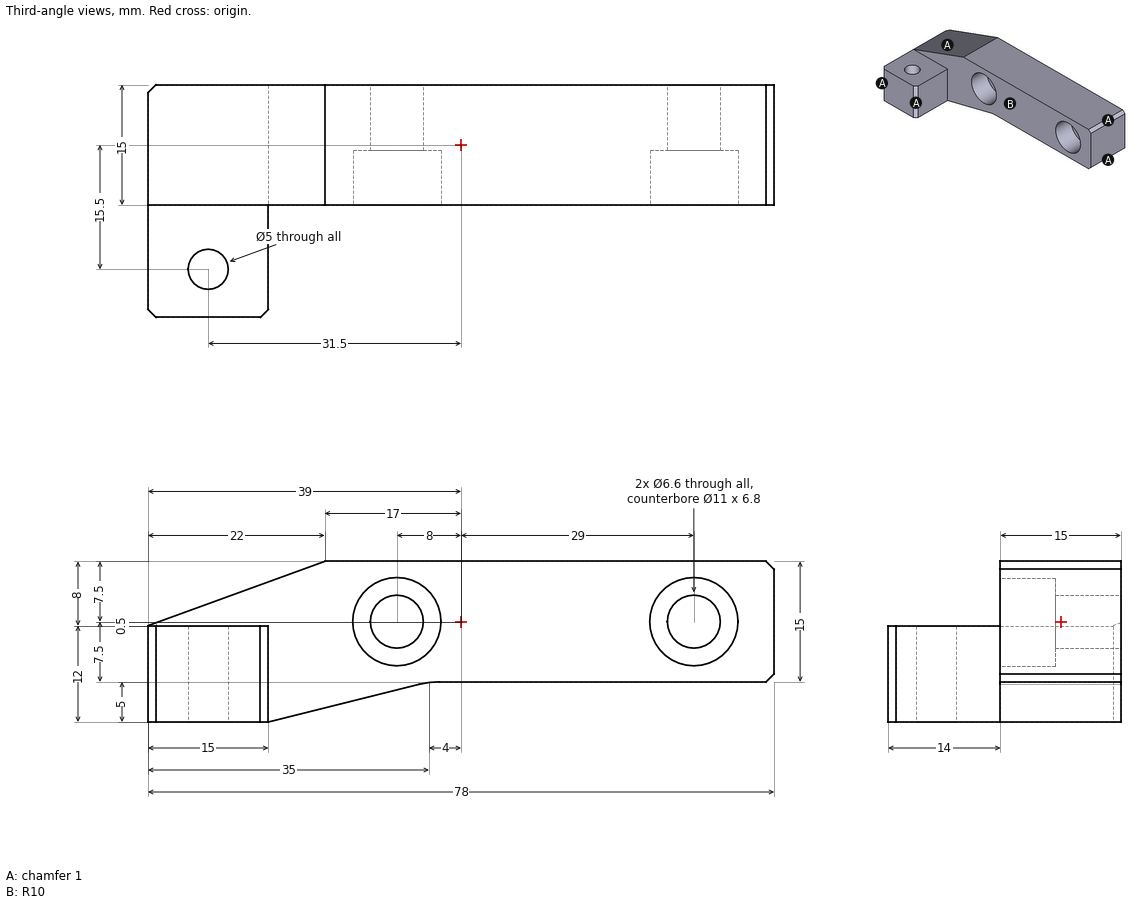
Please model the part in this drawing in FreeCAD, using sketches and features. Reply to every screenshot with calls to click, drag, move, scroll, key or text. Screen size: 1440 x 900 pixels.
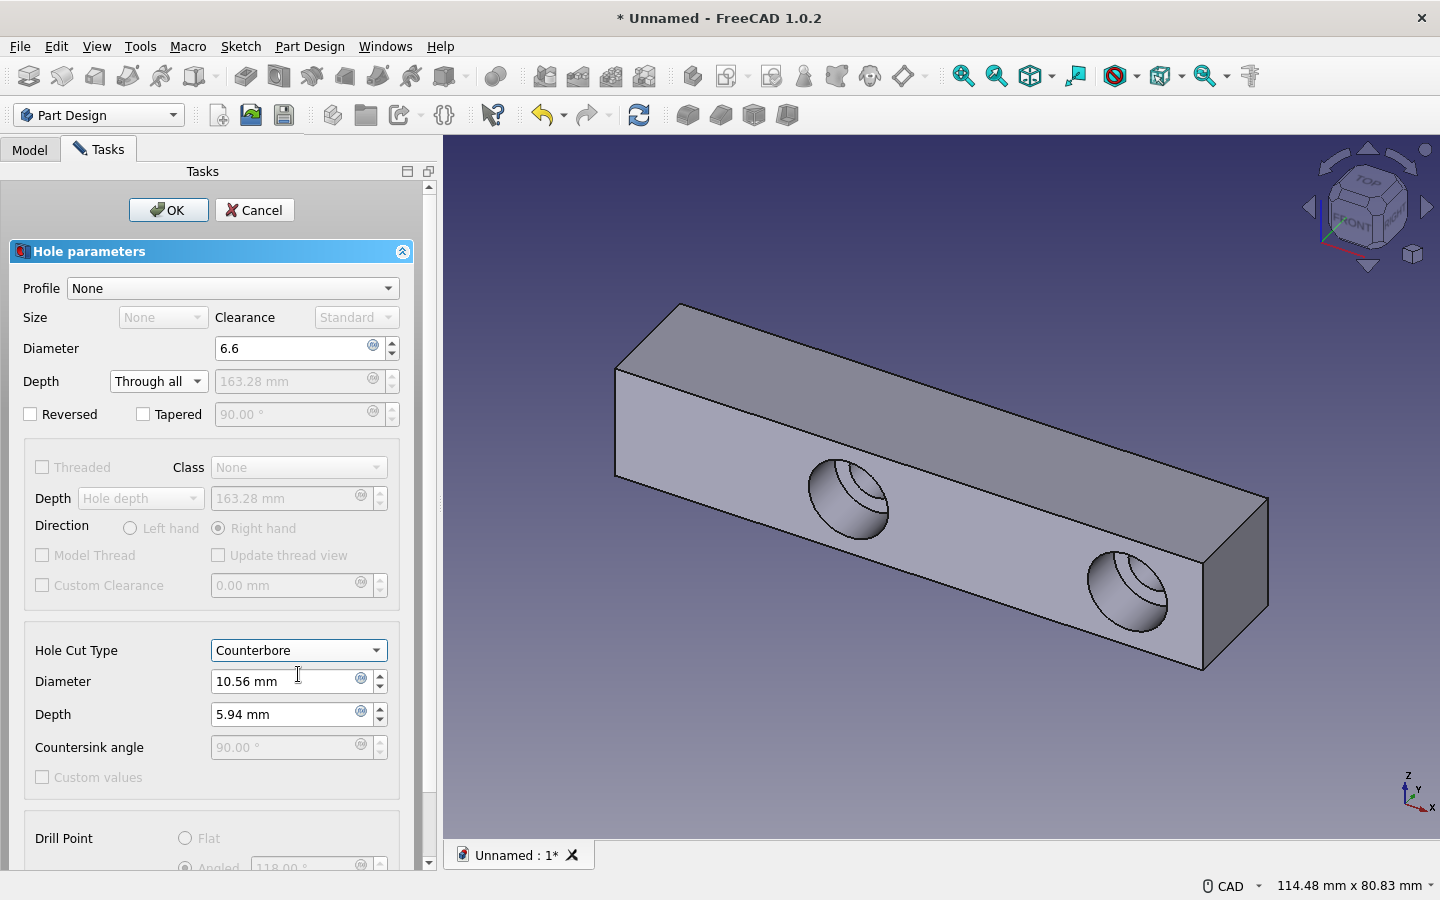
triple_click(292, 682)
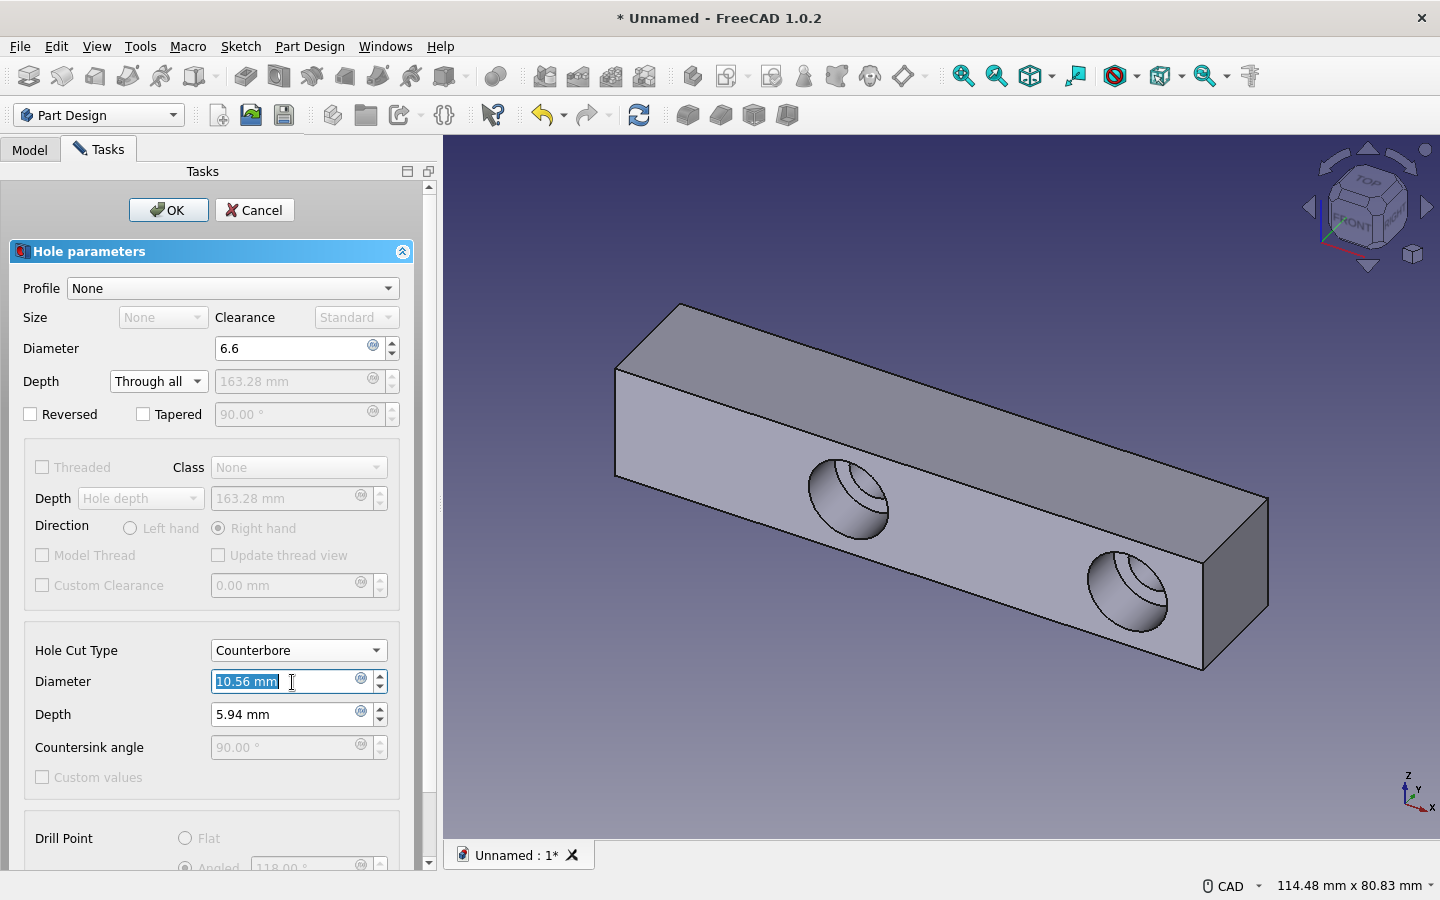
text(11)
key(Tab)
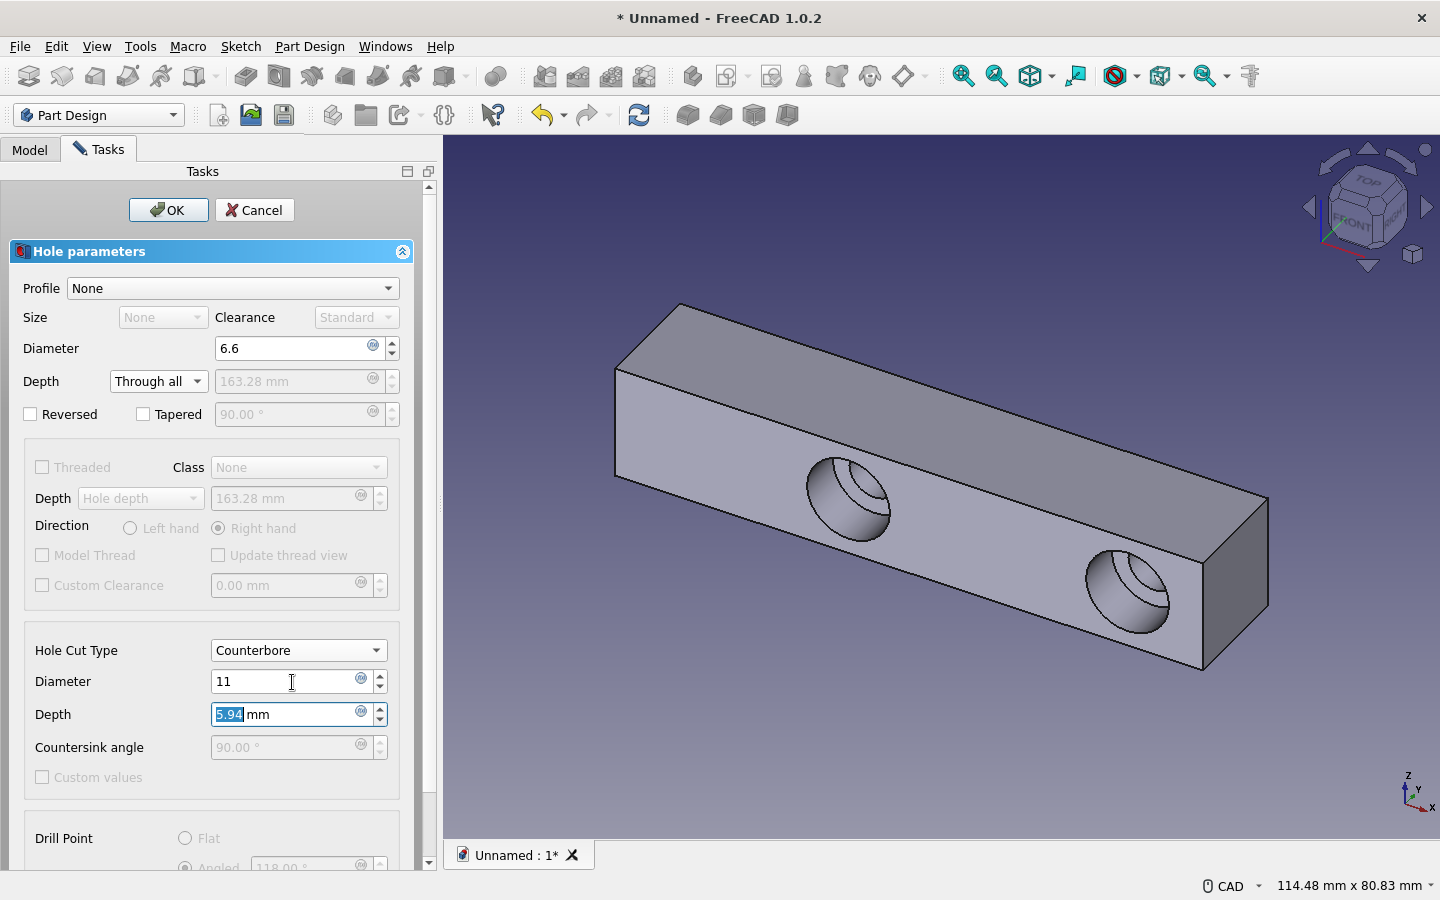
text(6.8)
key(Tab)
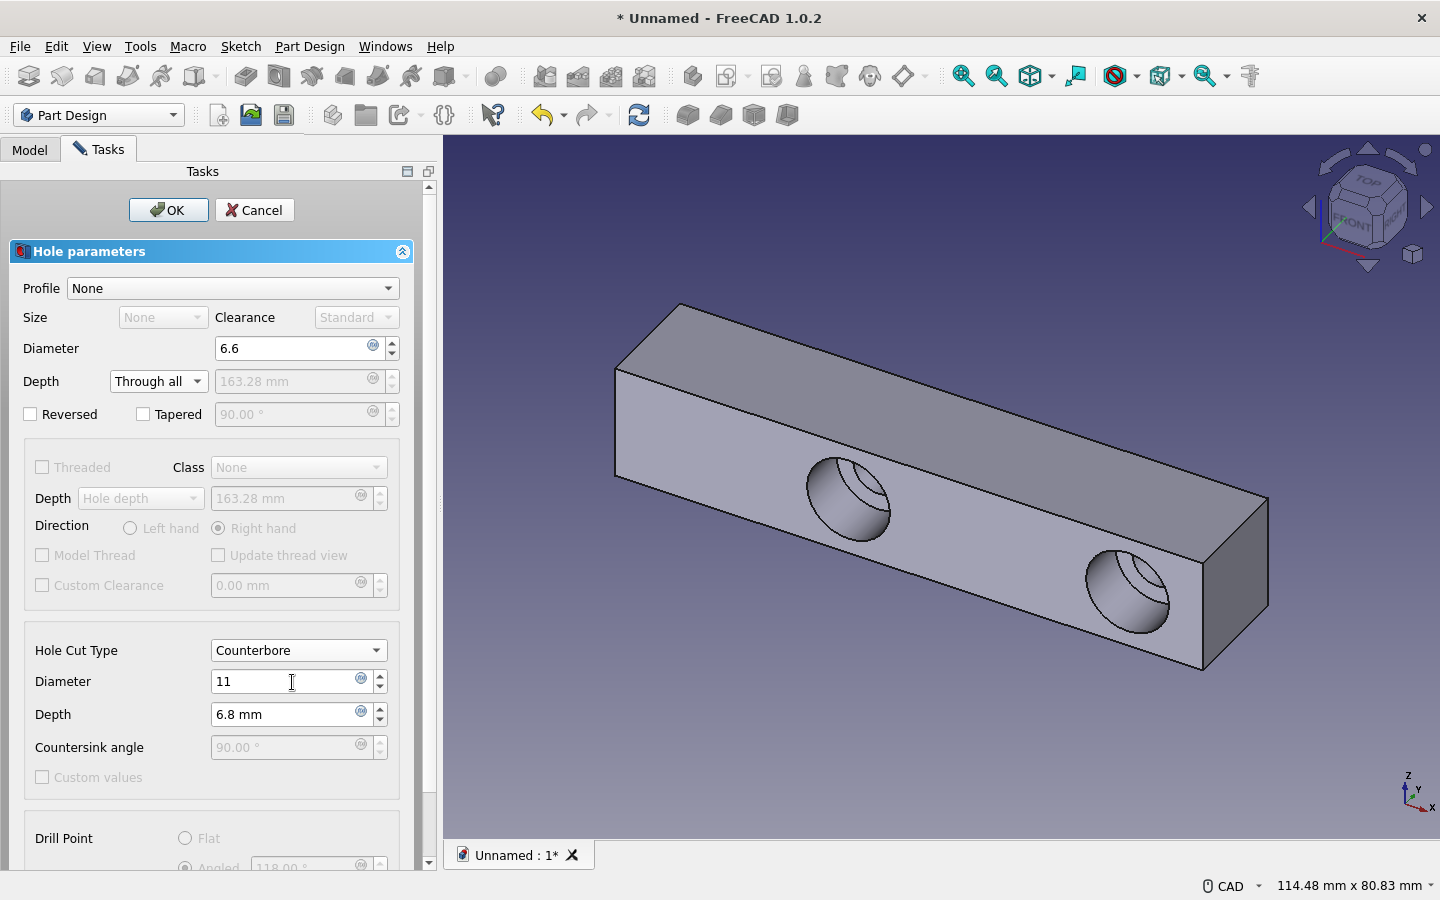
click(169, 210)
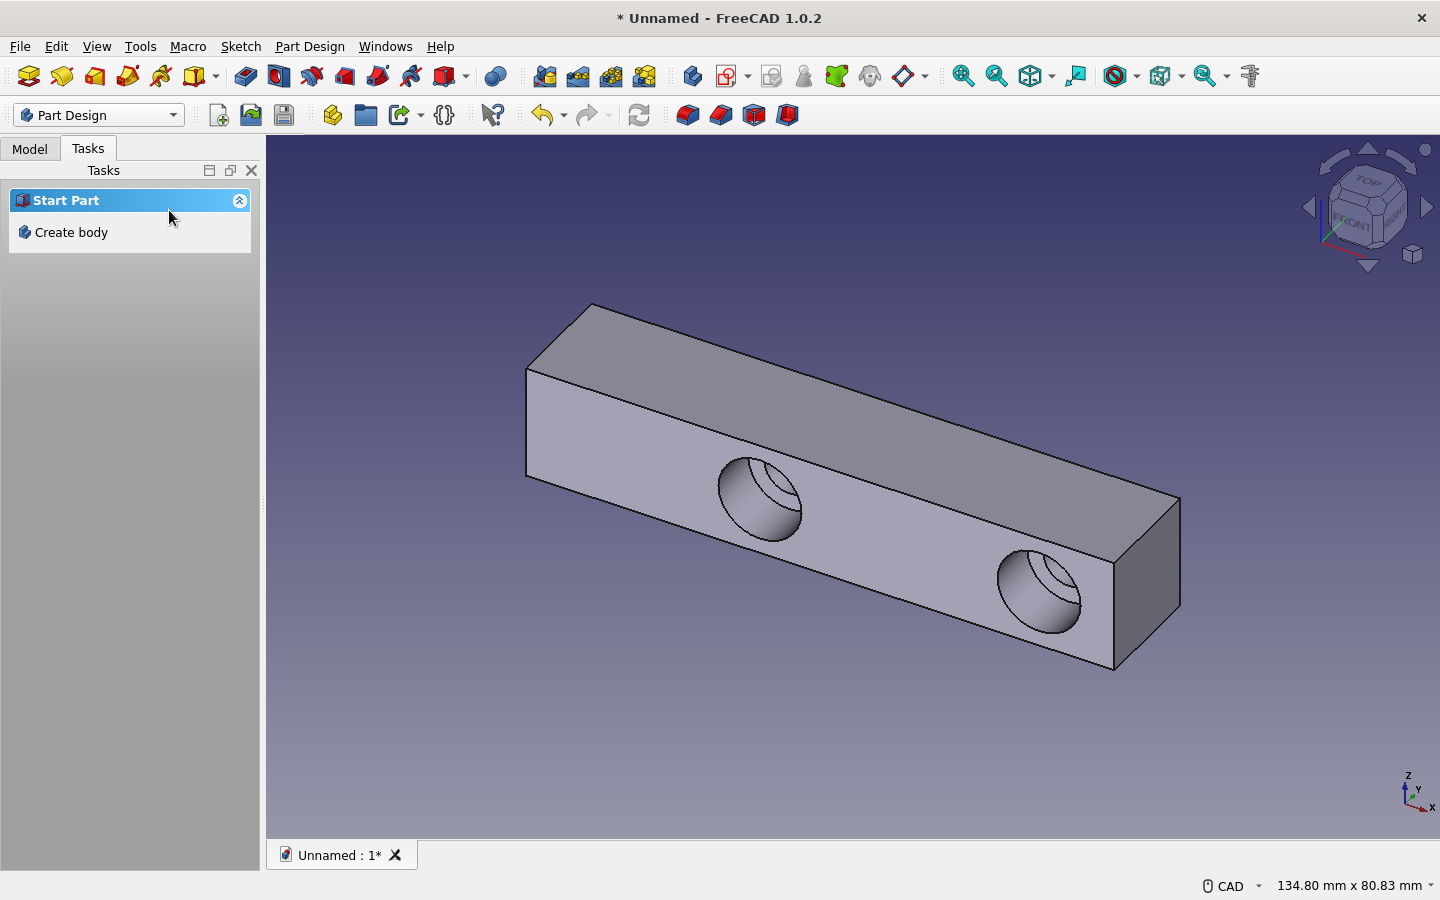
key(4)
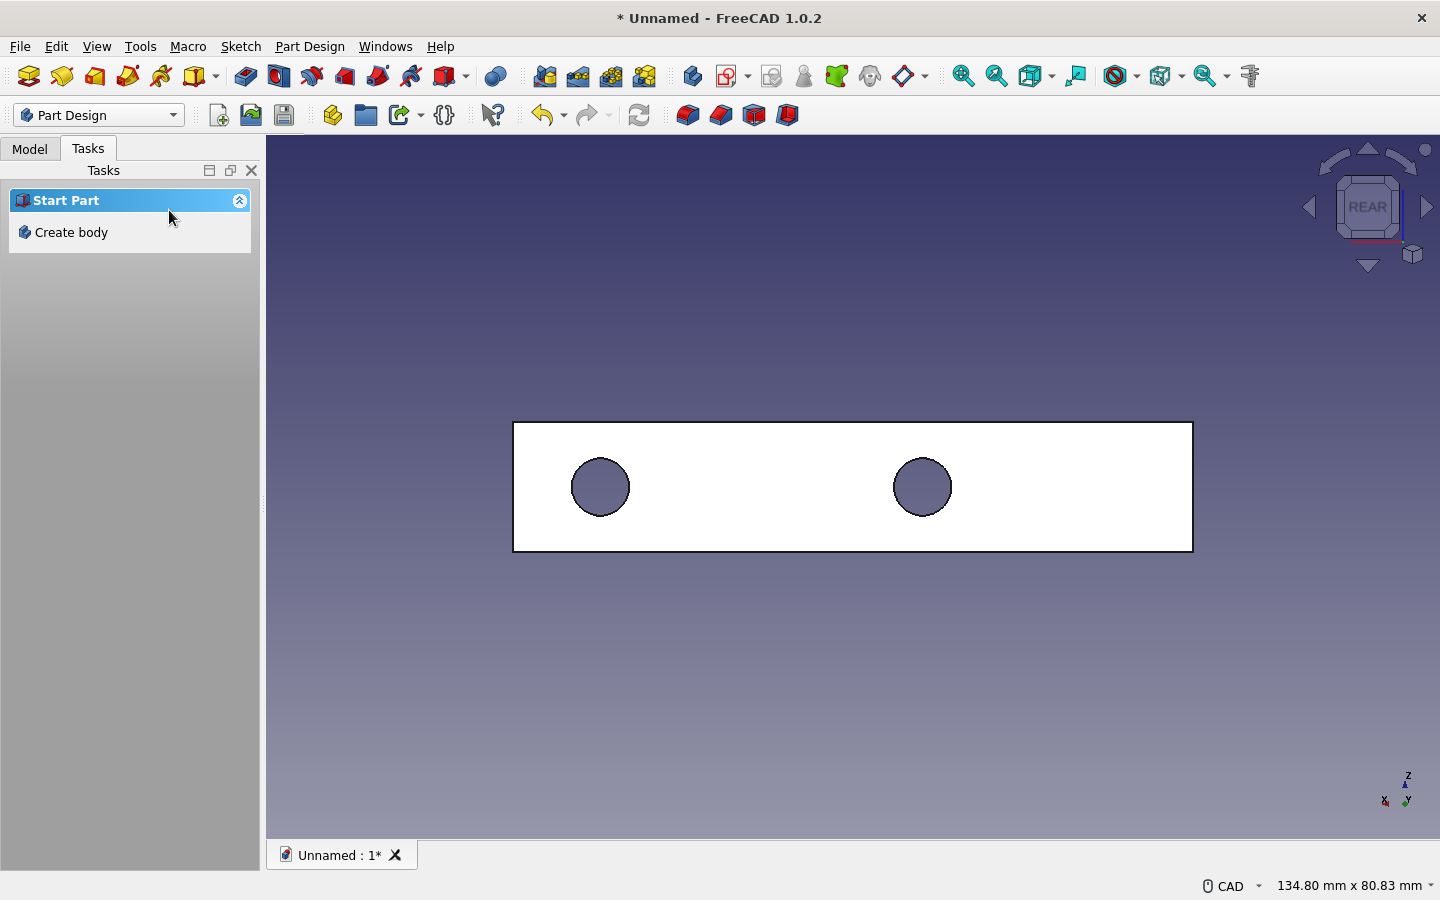
click(756, 486)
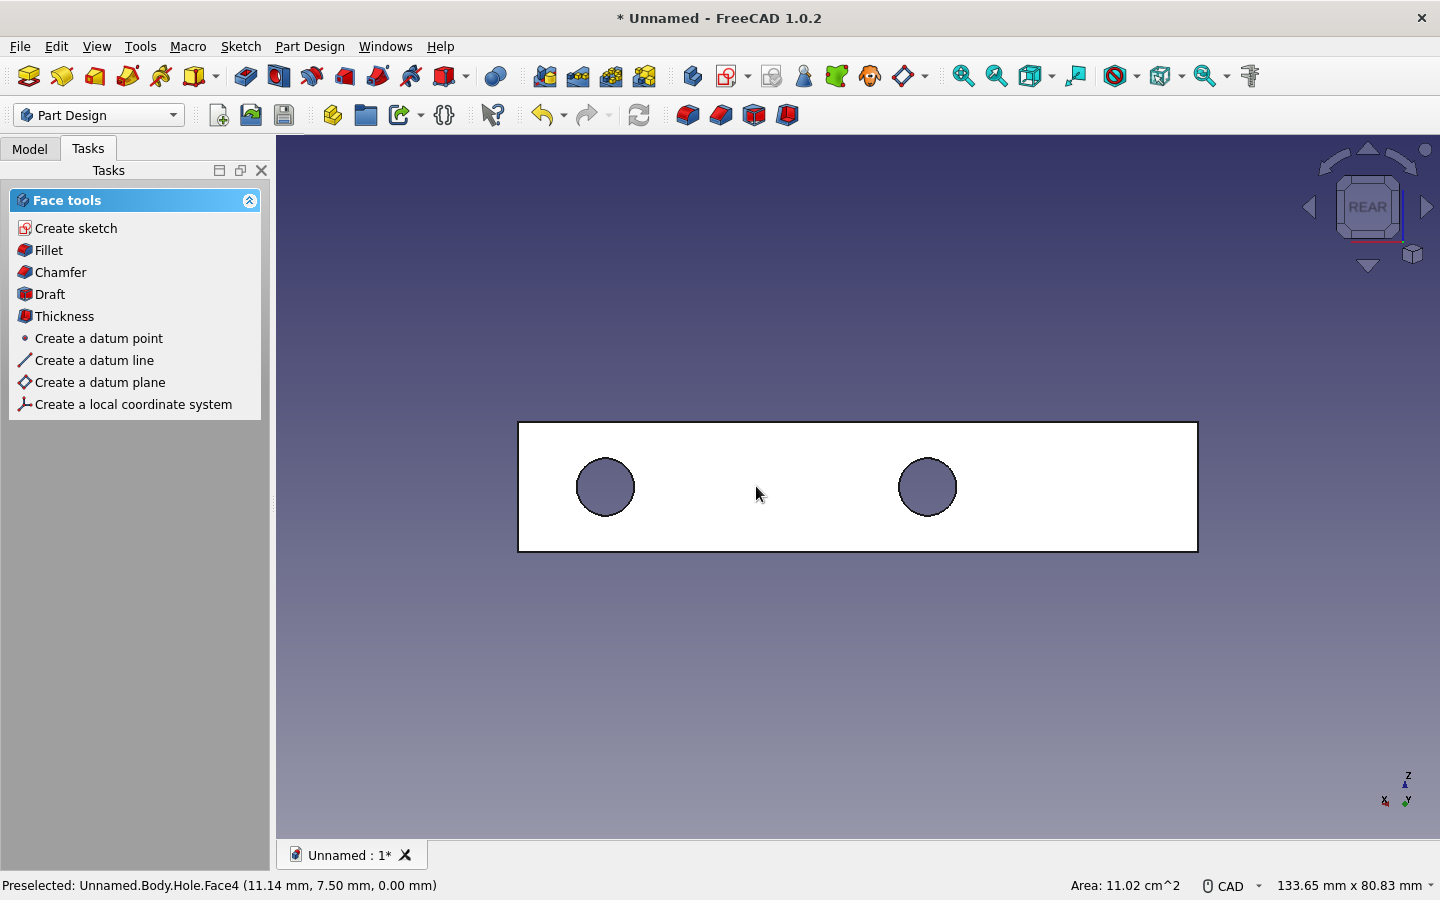
click(726, 76)